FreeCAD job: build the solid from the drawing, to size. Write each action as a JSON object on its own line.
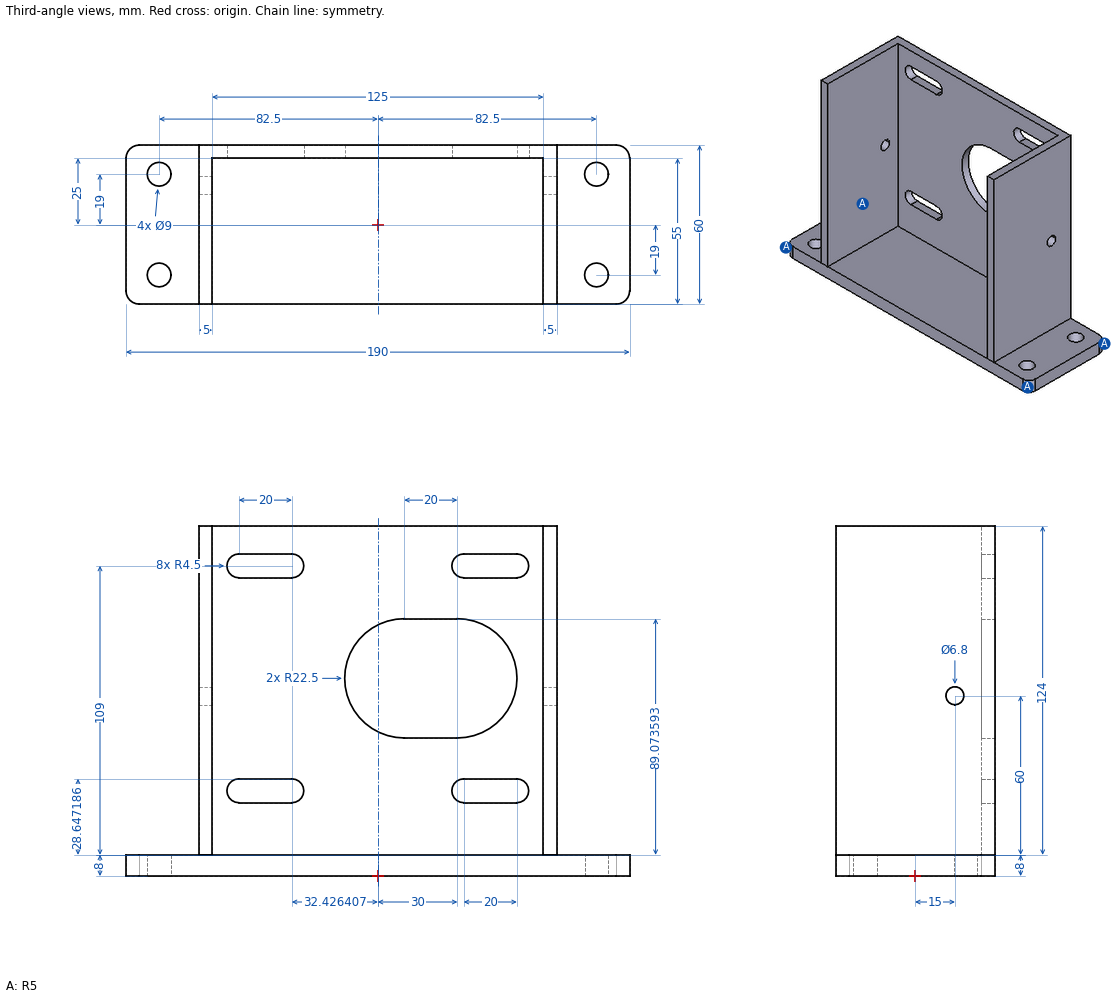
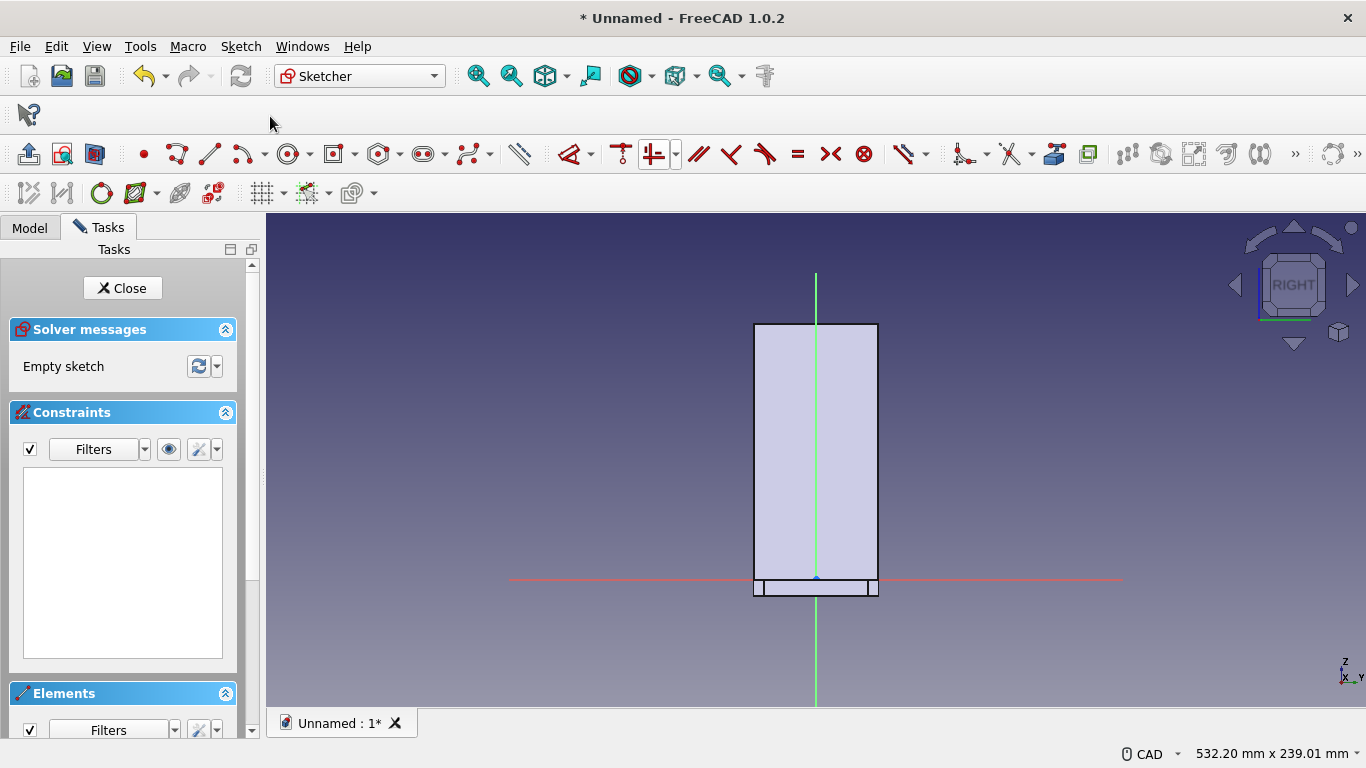
{"action": "scroll", "coordinate": [852, 456], "scroll_direction": "up", "scroll_amount": 15}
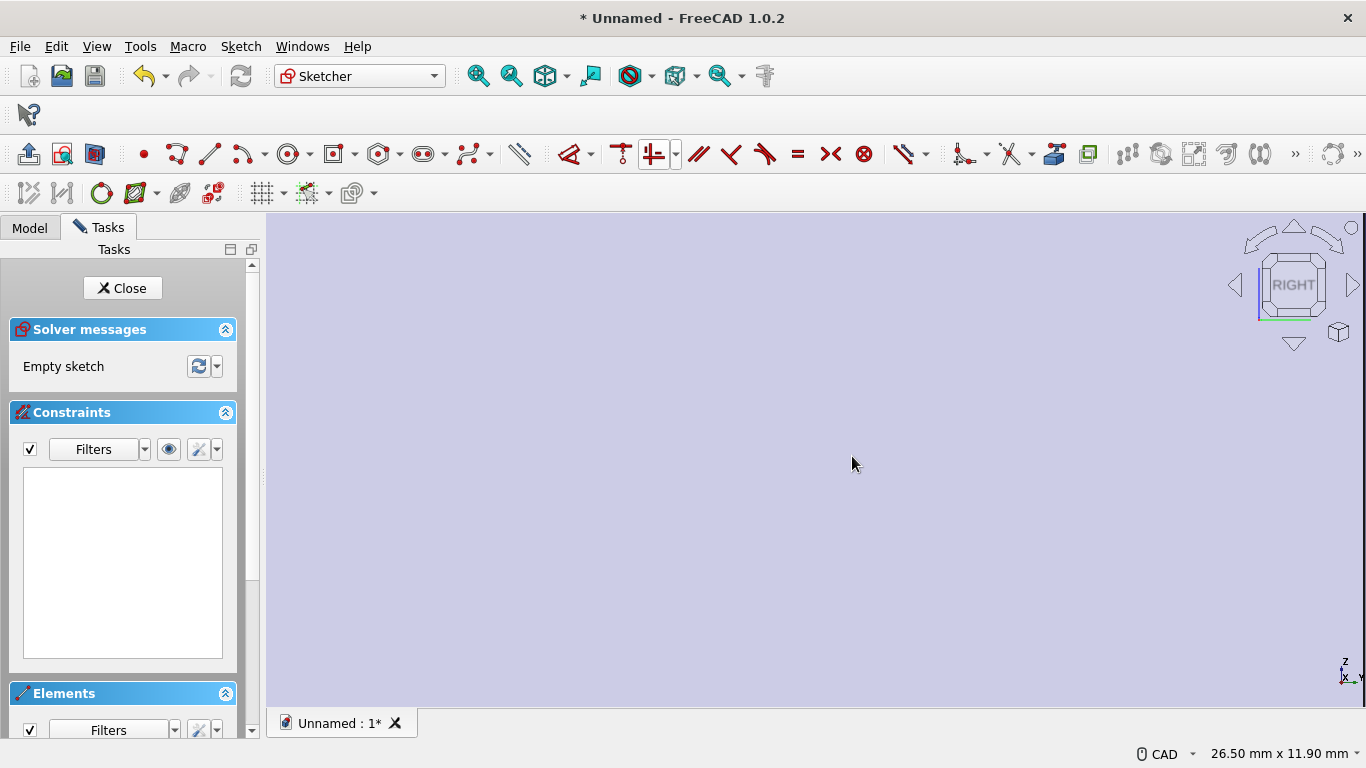
{"action": "left_click", "coordinate": [288, 154]}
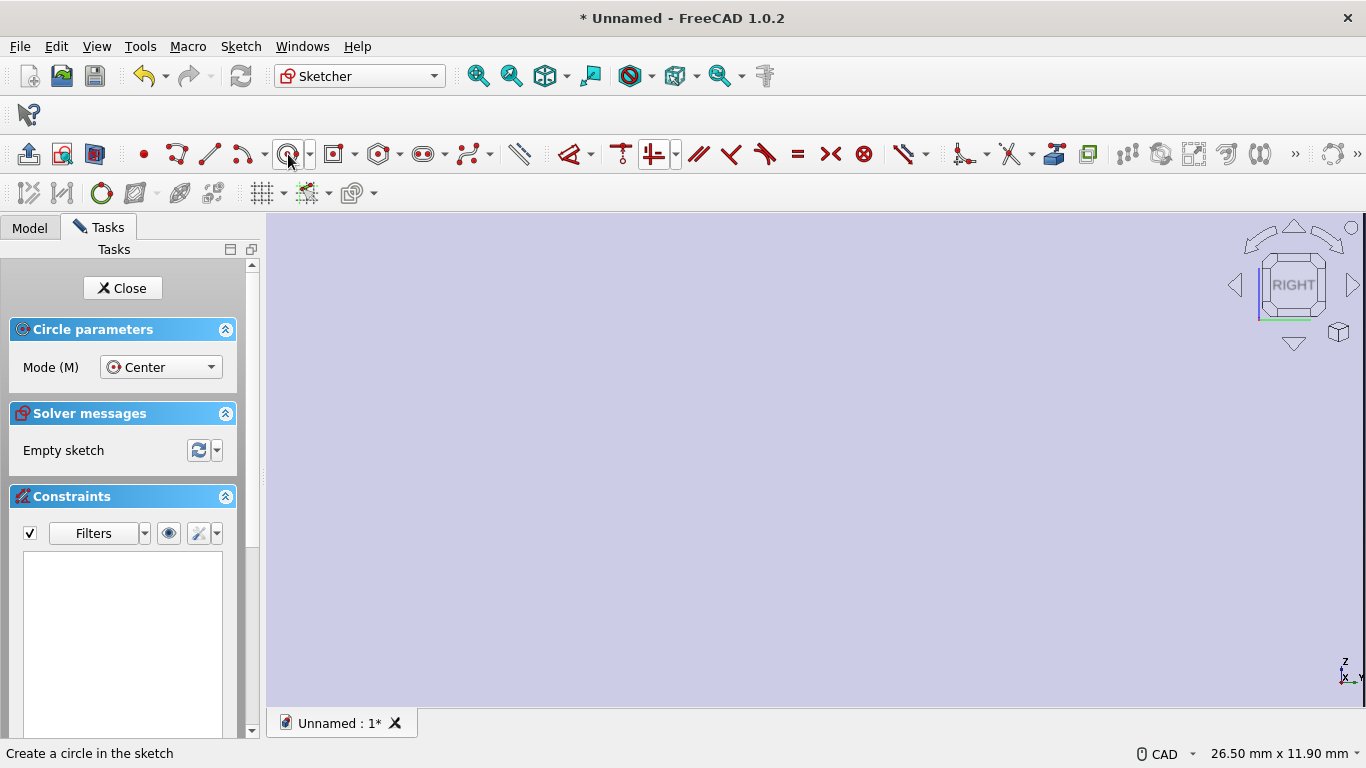
{"action": "left_click", "coordinate": [741, 444]}
{"action": "mouse_move", "coordinate": [841, 344]}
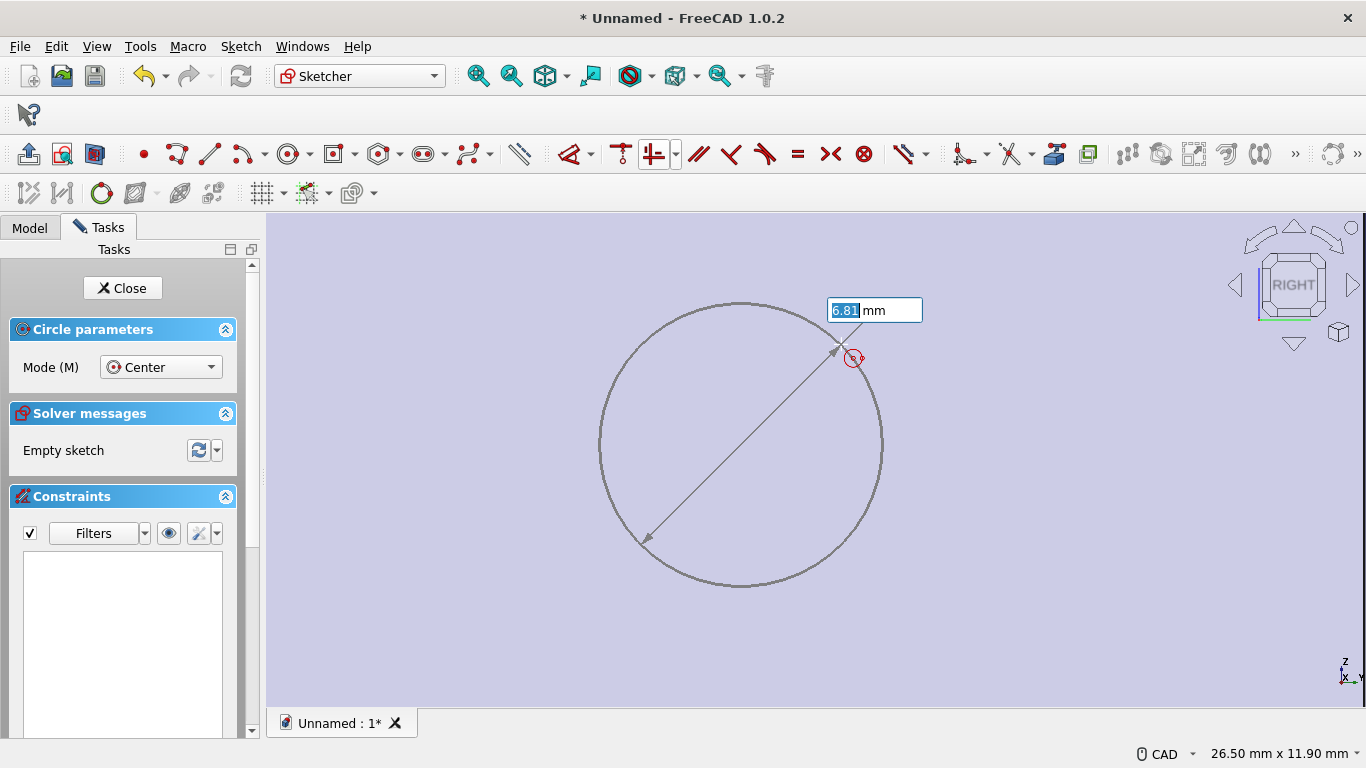
{"action": "type", "text": "6.8"}
{"action": "key", "text": "Return"}
{"action": "key", "text": "Escape"}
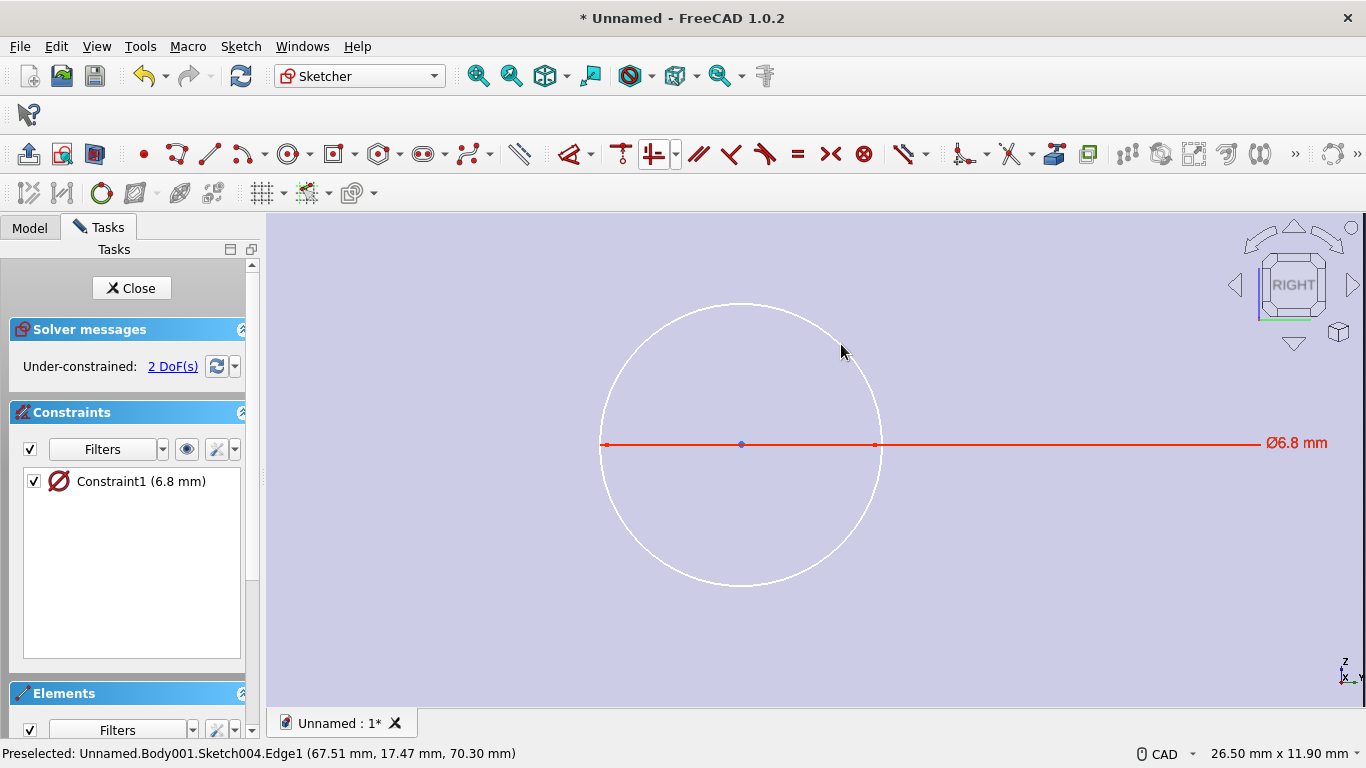
{"action": "left_click", "coordinate": [568, 154]}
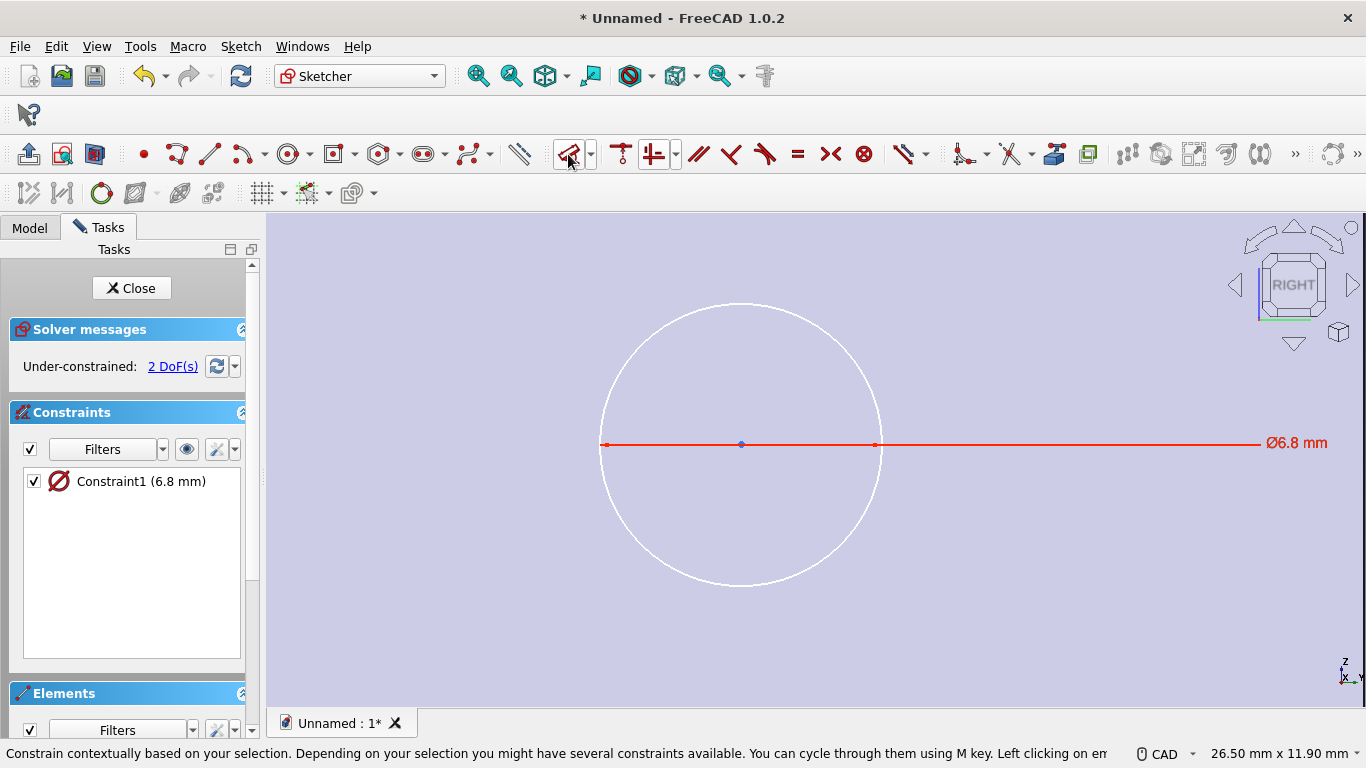
{"action": "left_click", "coordinate": [741, 445]}
{"action": "left_click", "coordinate": [518, 411]}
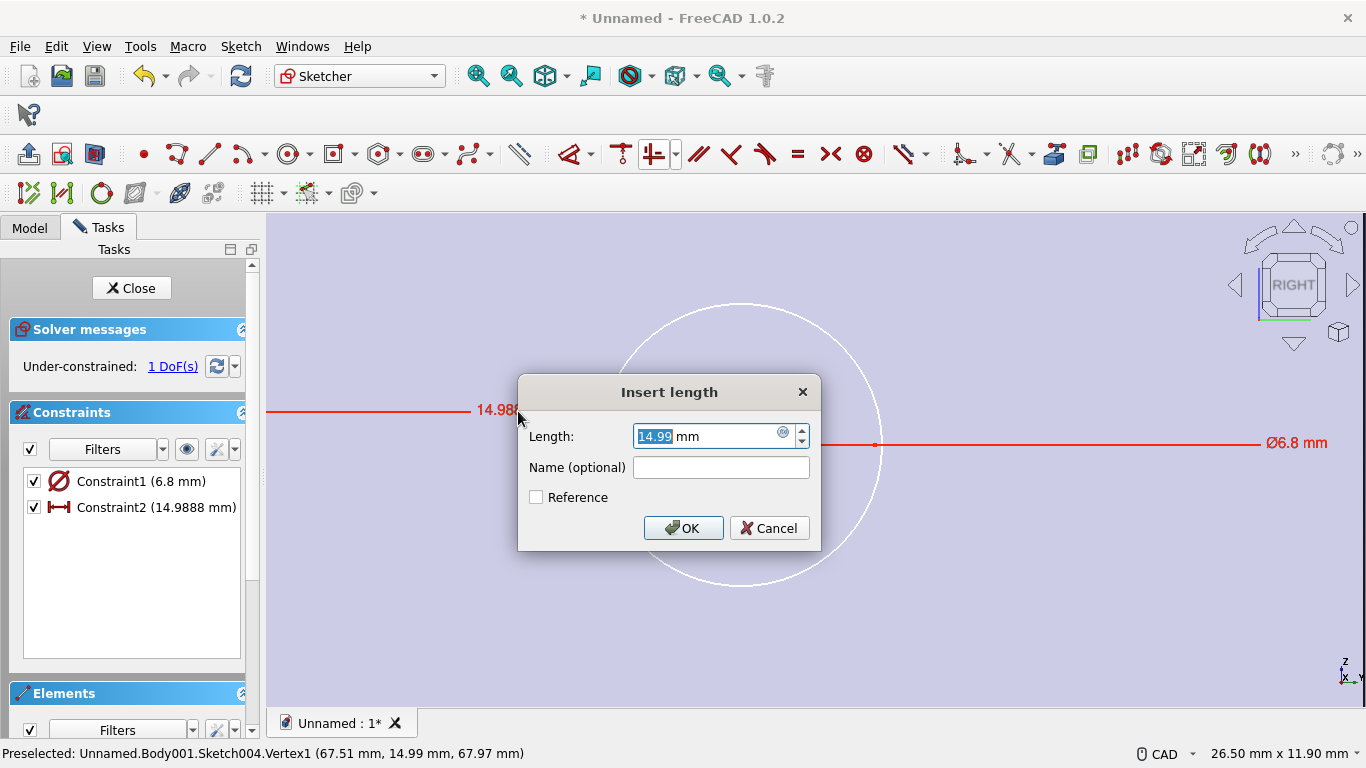
{"action": "type", "text": "15"}
{"action": "key", "text": "Return"}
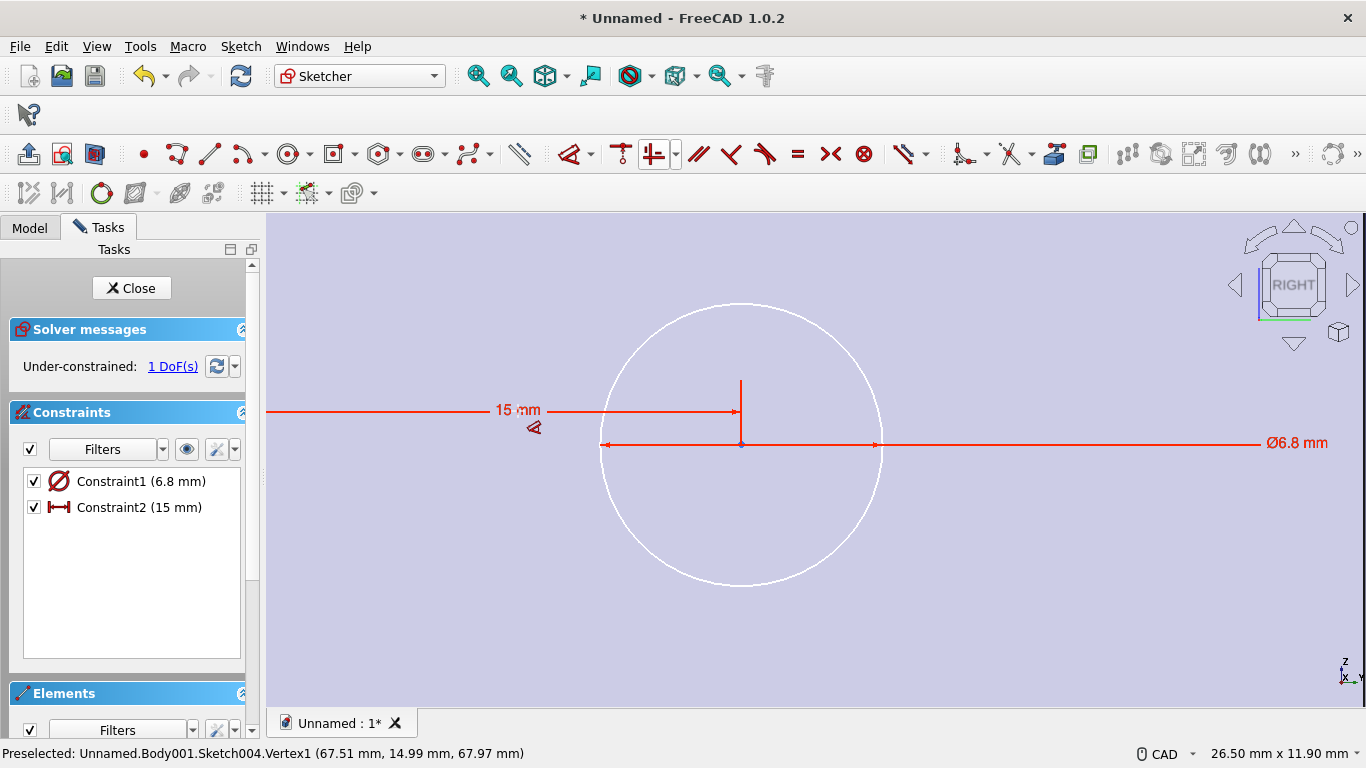
{"action": "left_click", "coordinate": [741, 445]}
{"action": "left_click", "coordinate": [775, 562]}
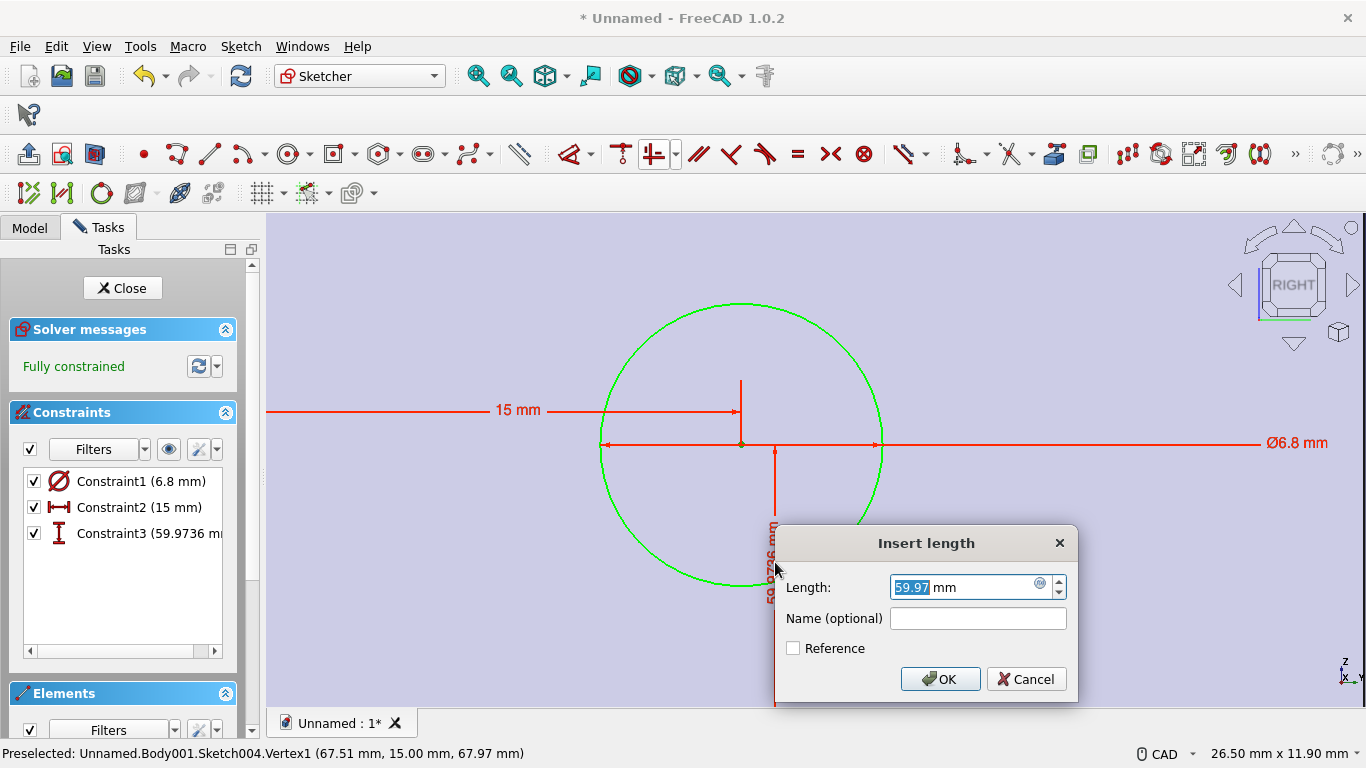
{"action": "type", "text": "60"}
{"action": "key", "text": "Return"}
{"action": "key", "text": "Escape"}